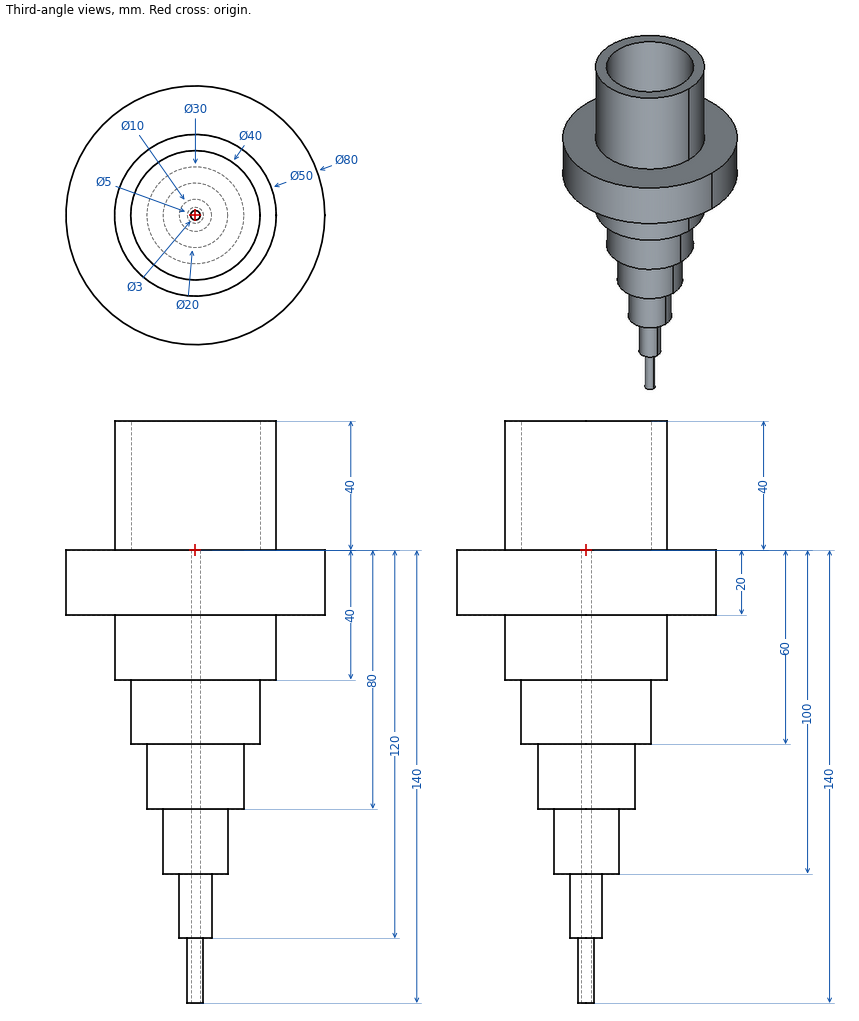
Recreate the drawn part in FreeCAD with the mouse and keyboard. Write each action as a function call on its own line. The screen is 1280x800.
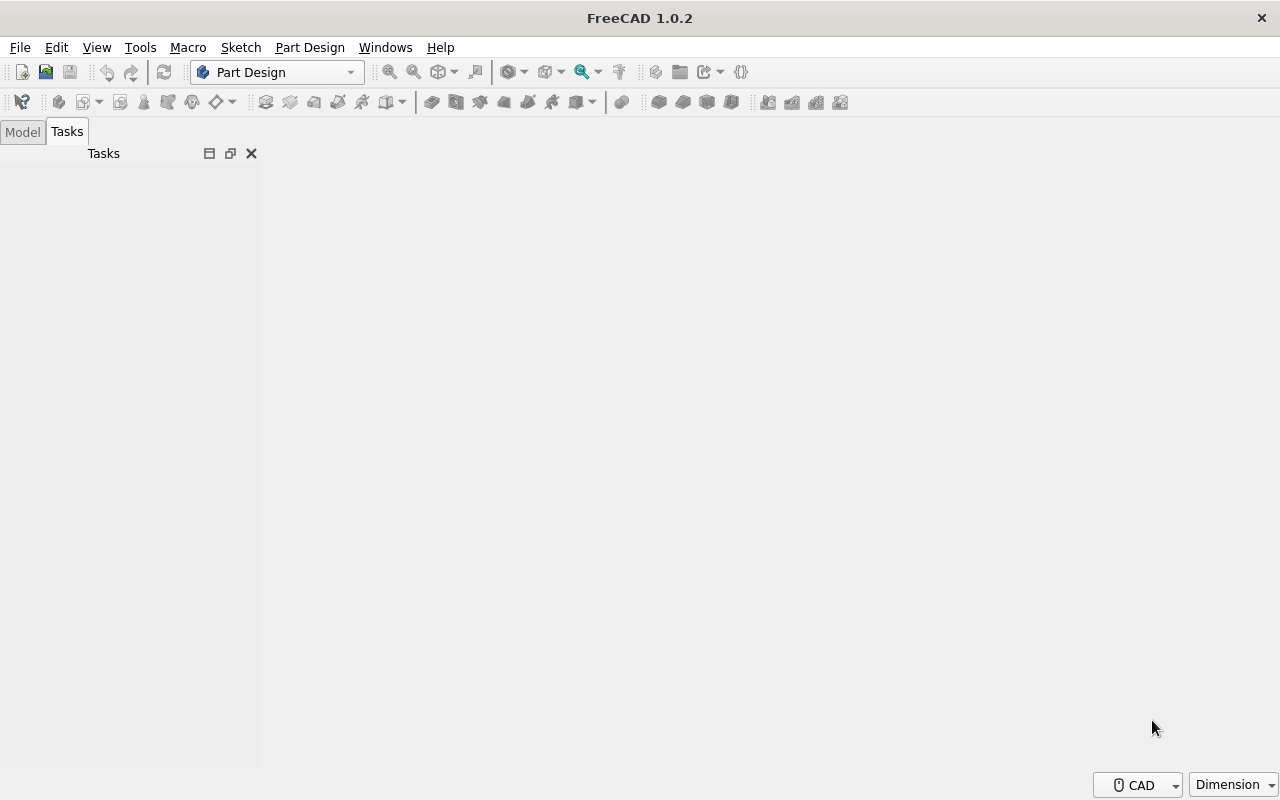
key(ctrl+n)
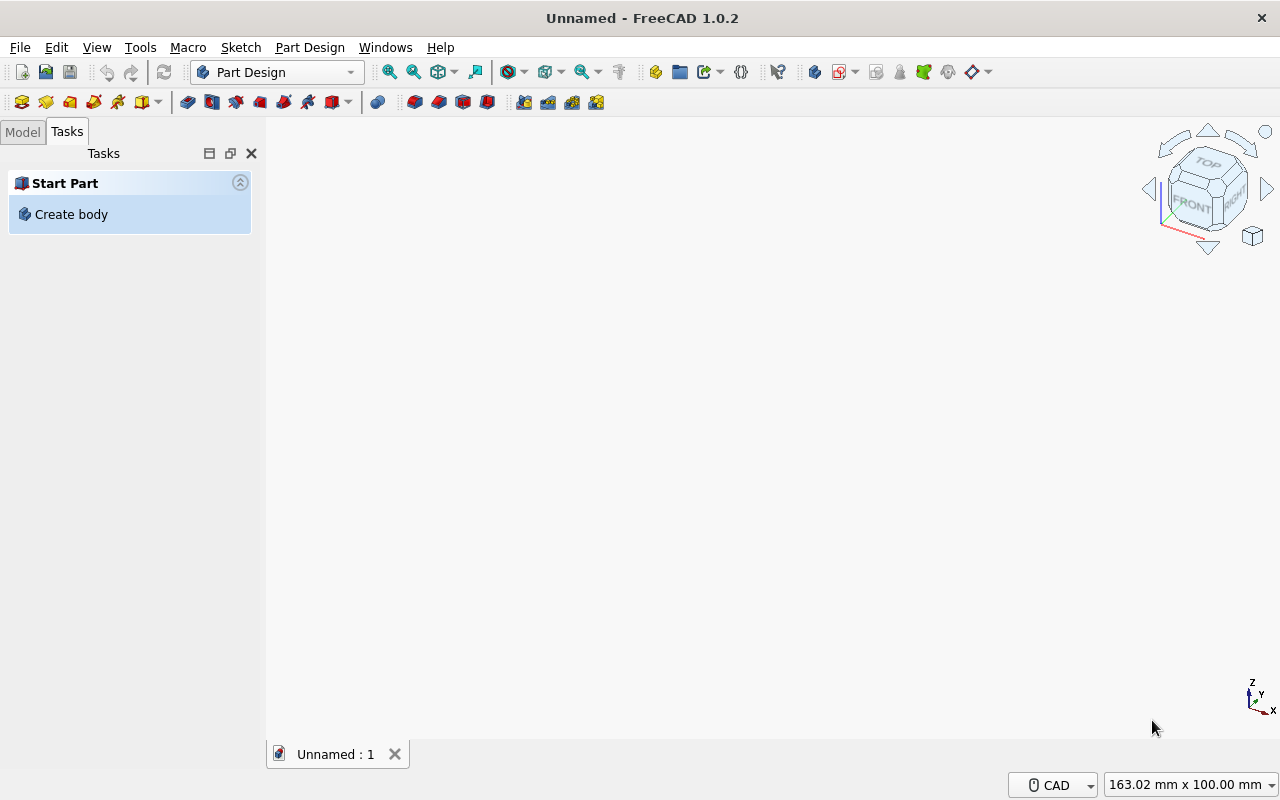
click(840, 72)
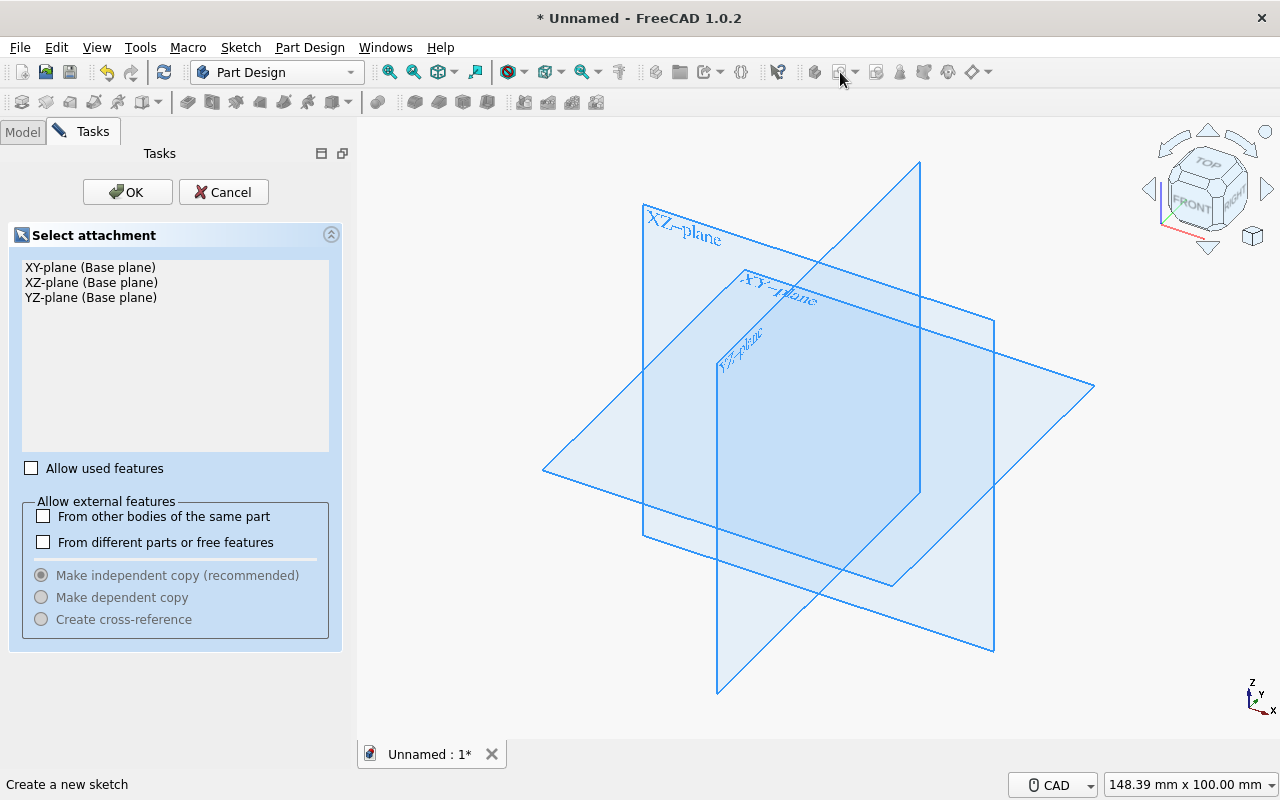
click(82, 268)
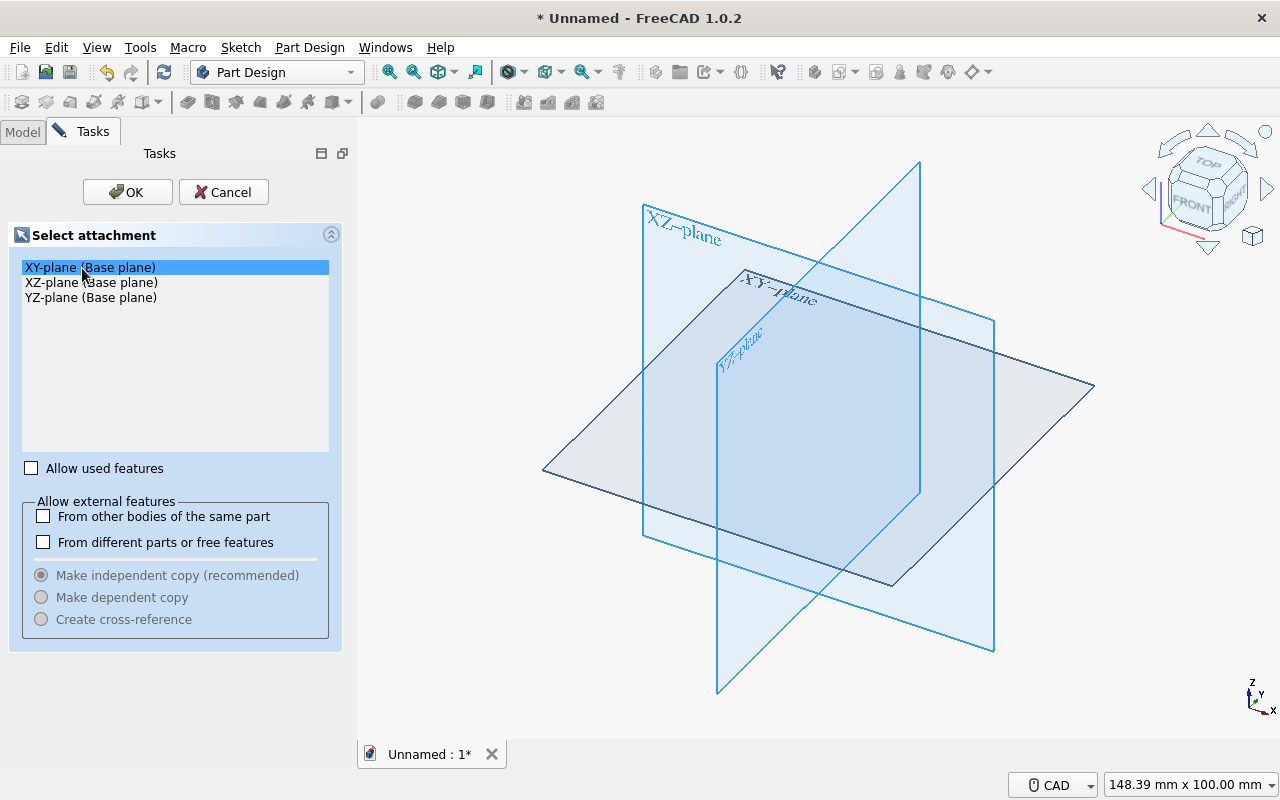
click(128, 192)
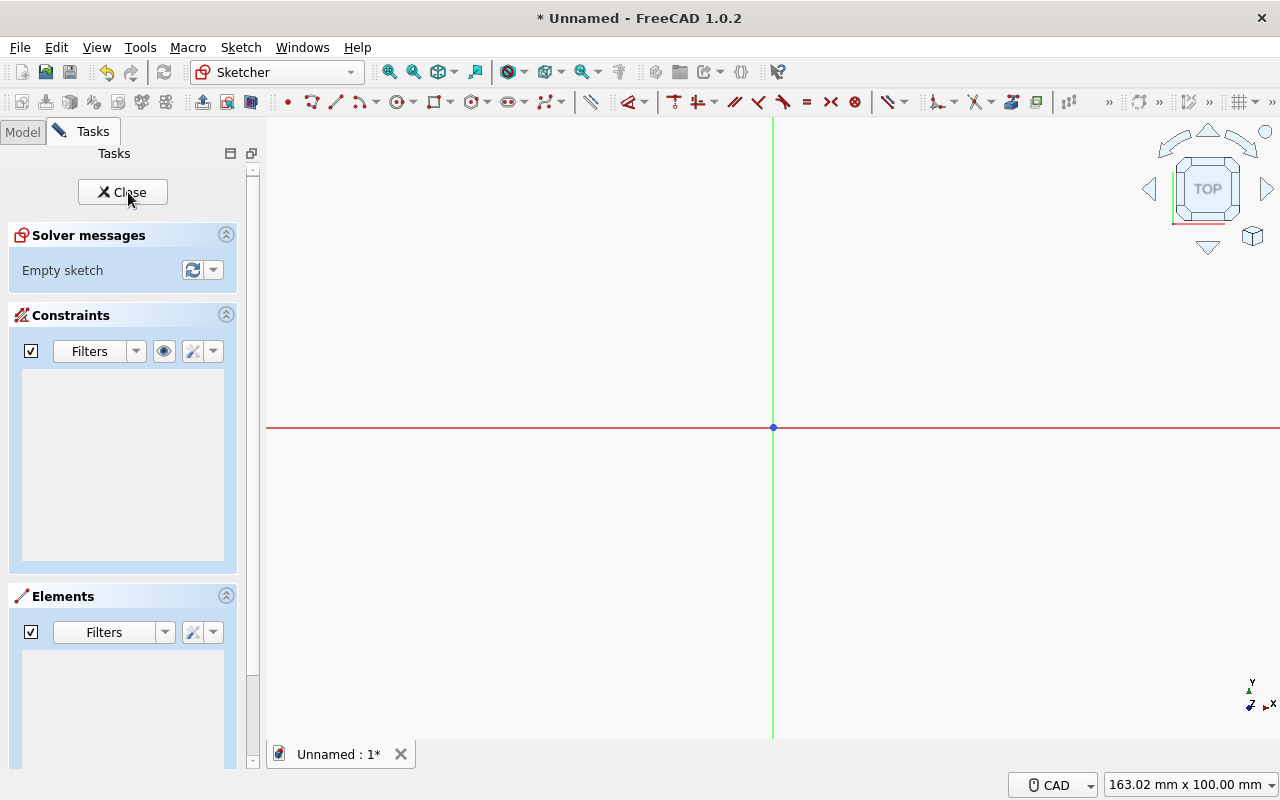
key(g)
key(c)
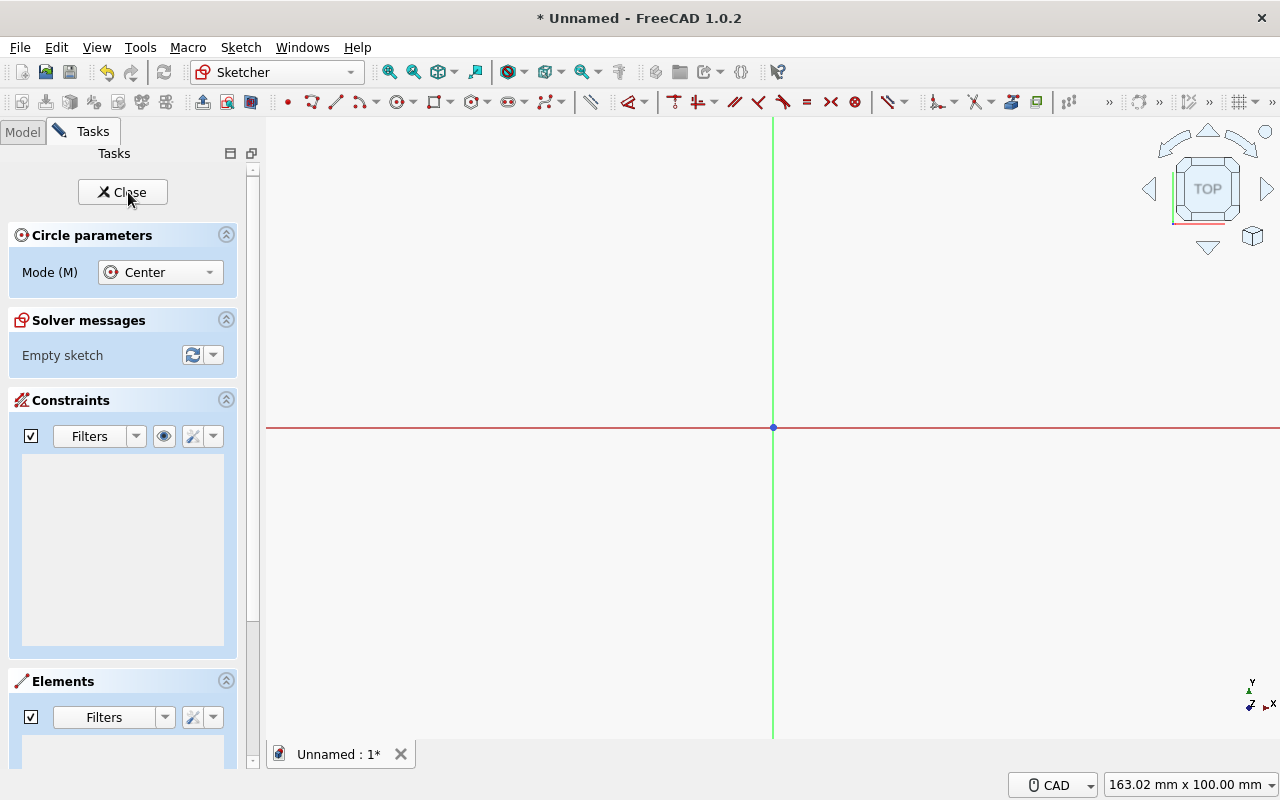
click(773, 428)
move(949, 252)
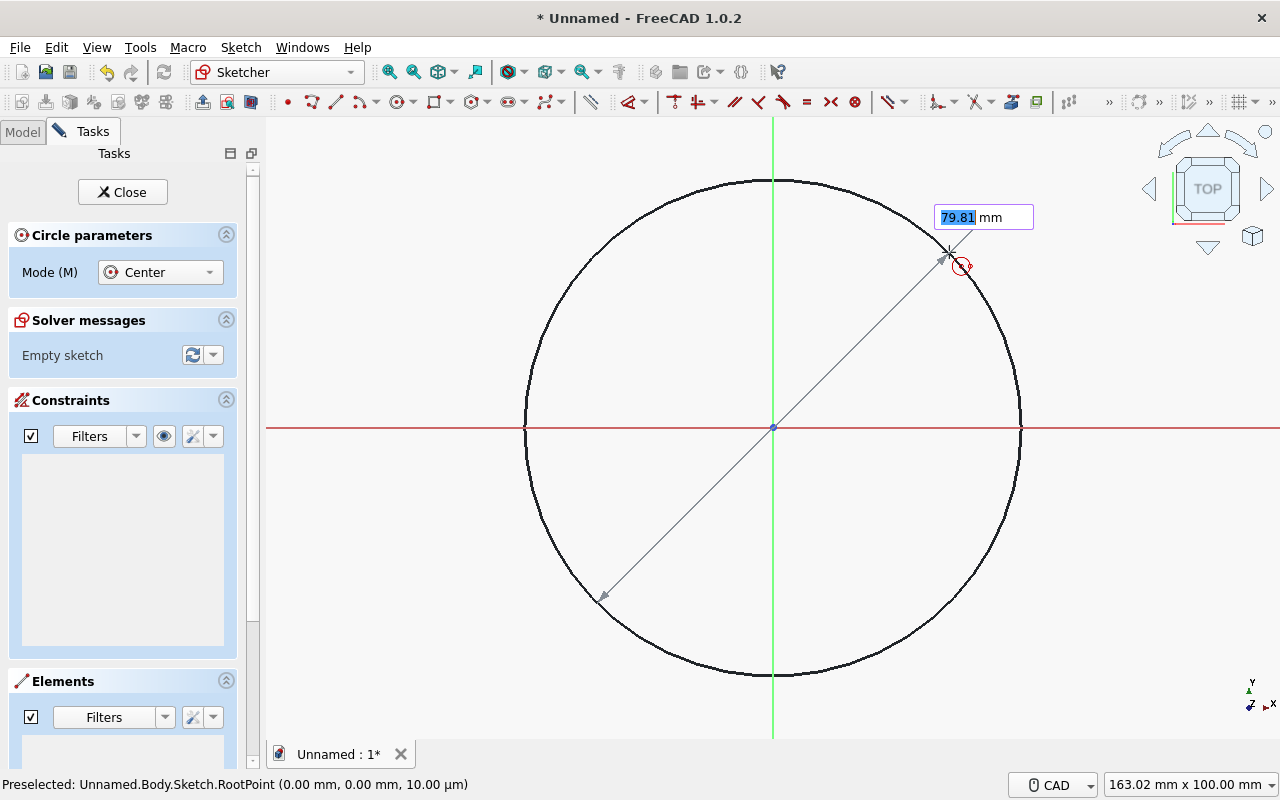
text(80)
key(Return)
key(Escape)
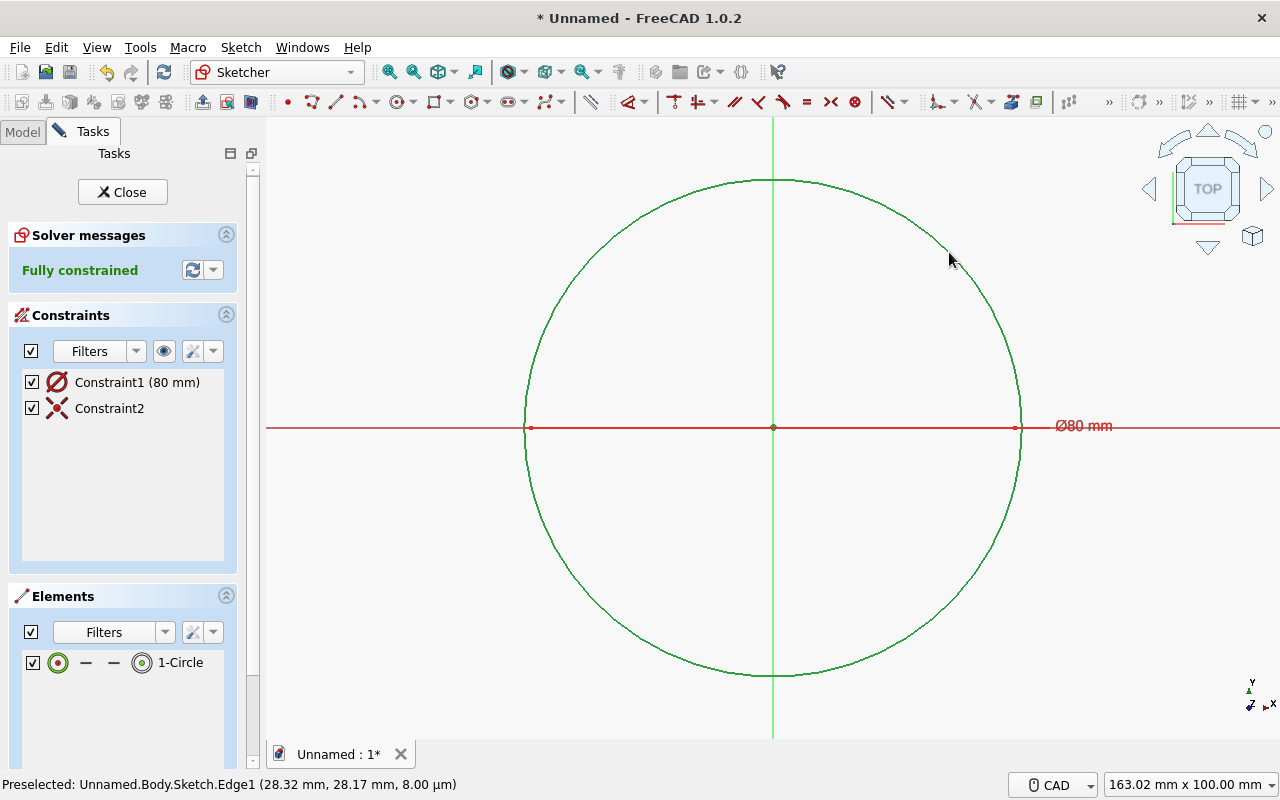
click(123, 192)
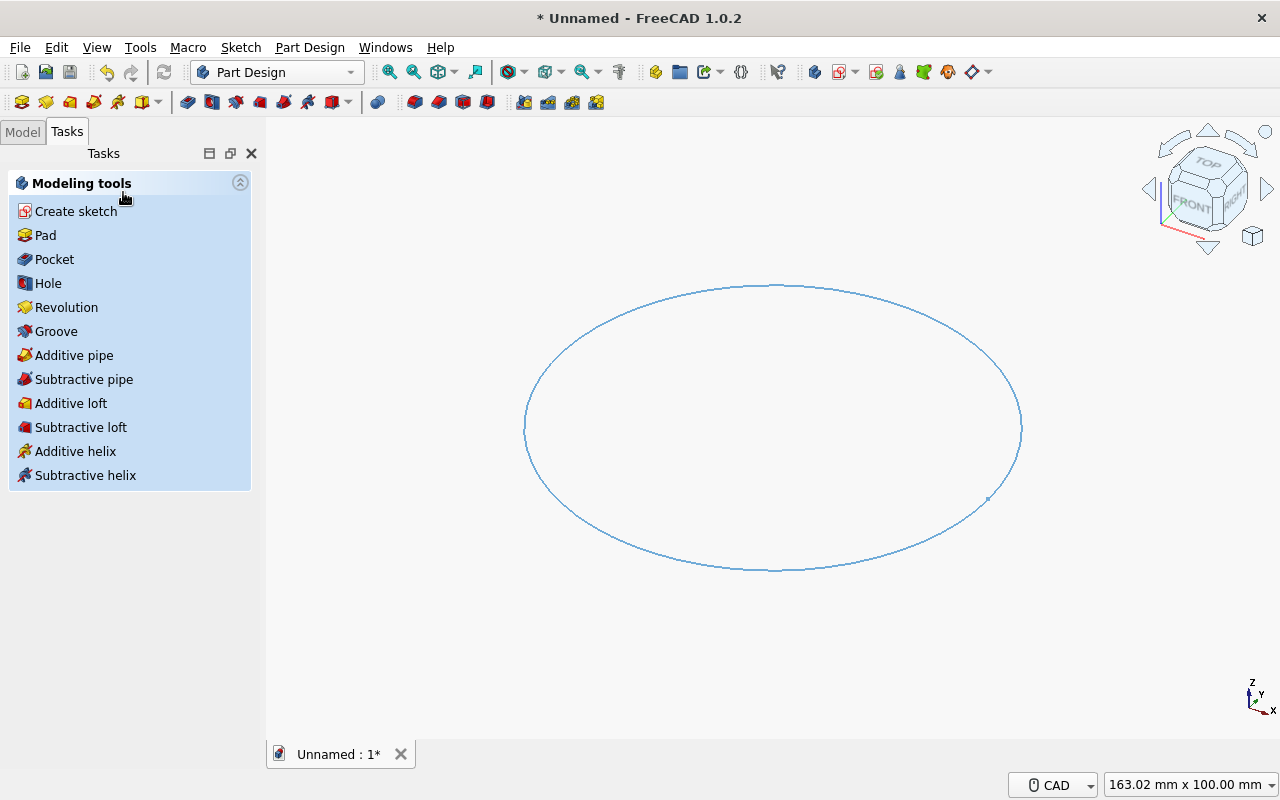
click(22, 102)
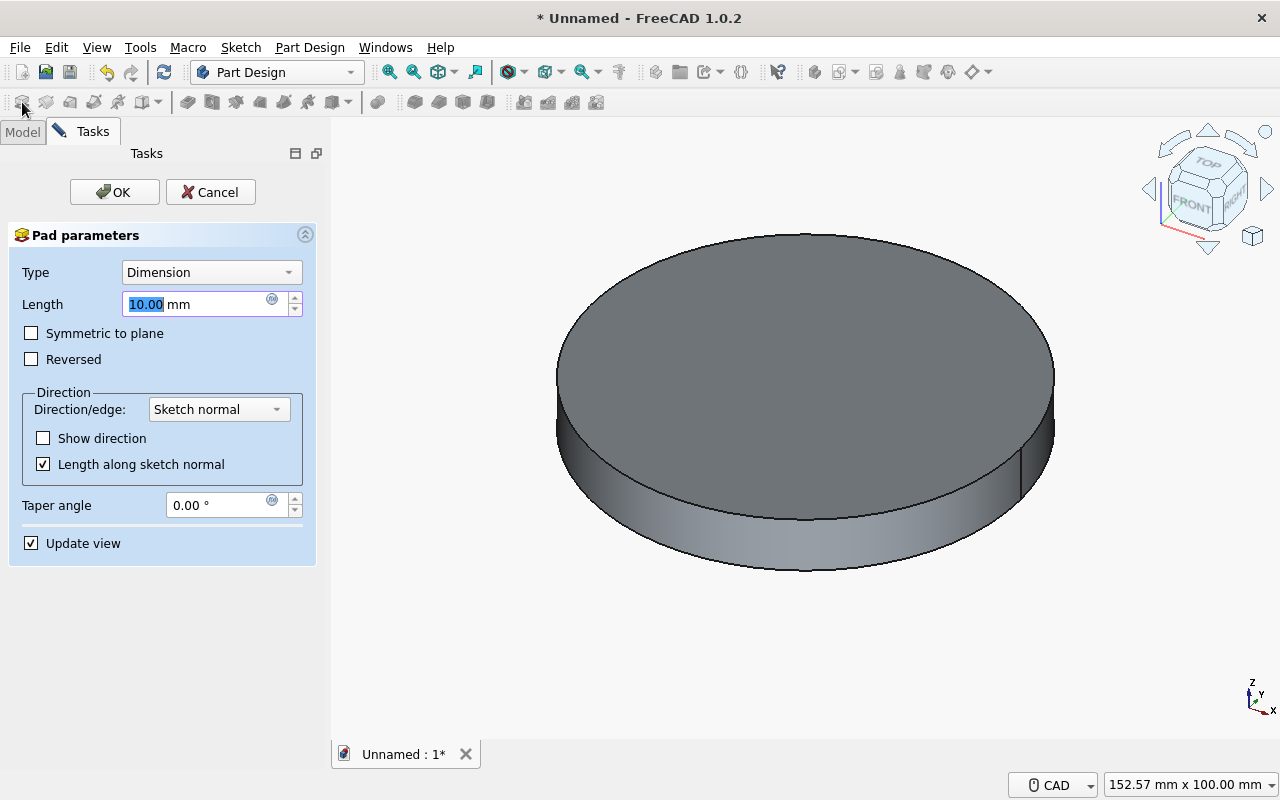
text(20)
key(Tab)